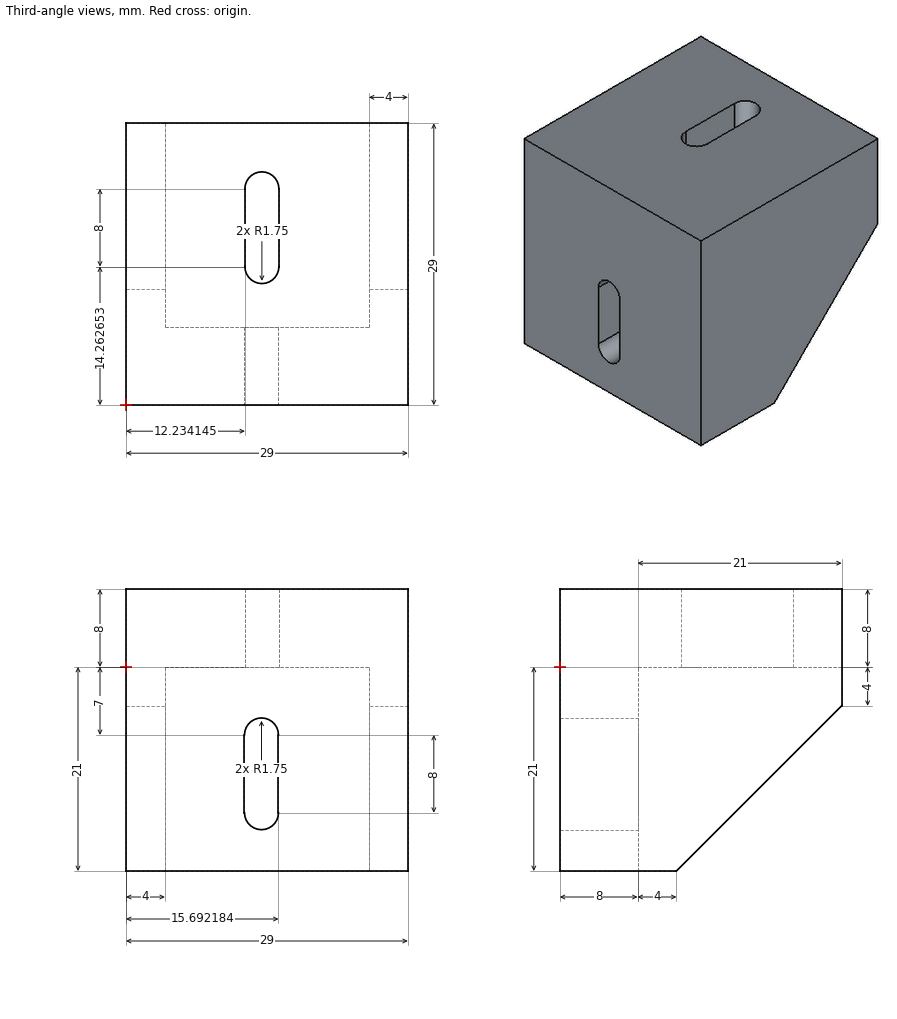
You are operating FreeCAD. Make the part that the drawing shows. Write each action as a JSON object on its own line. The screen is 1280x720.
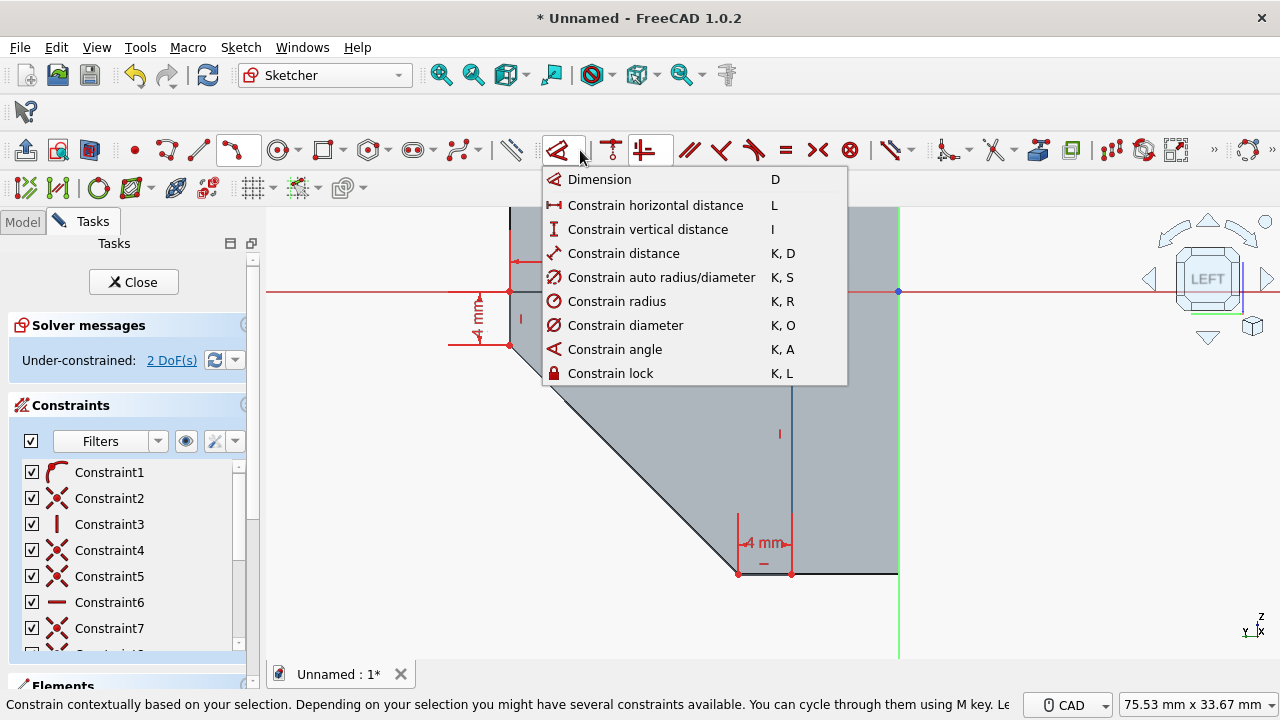
{"action": "left_click", "coordinate": [695, 229]}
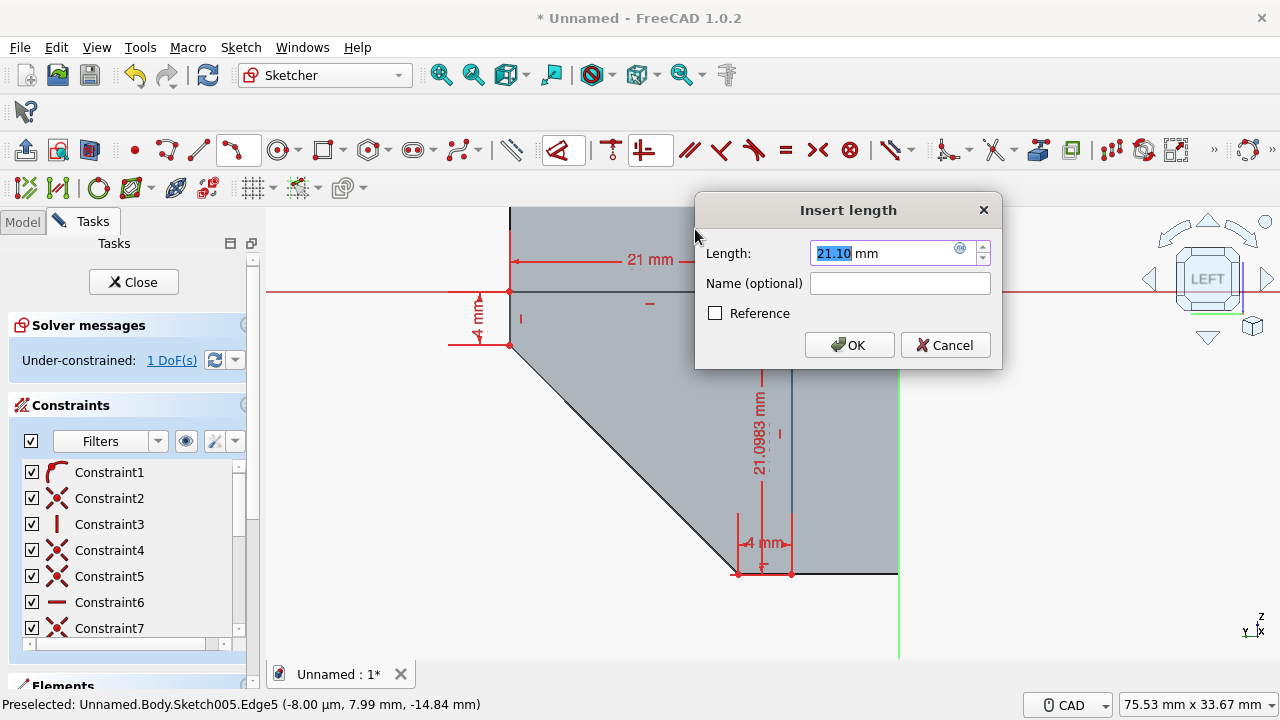
{"action": "type", "text": "21"}
{"action": "key", "text": "Return"}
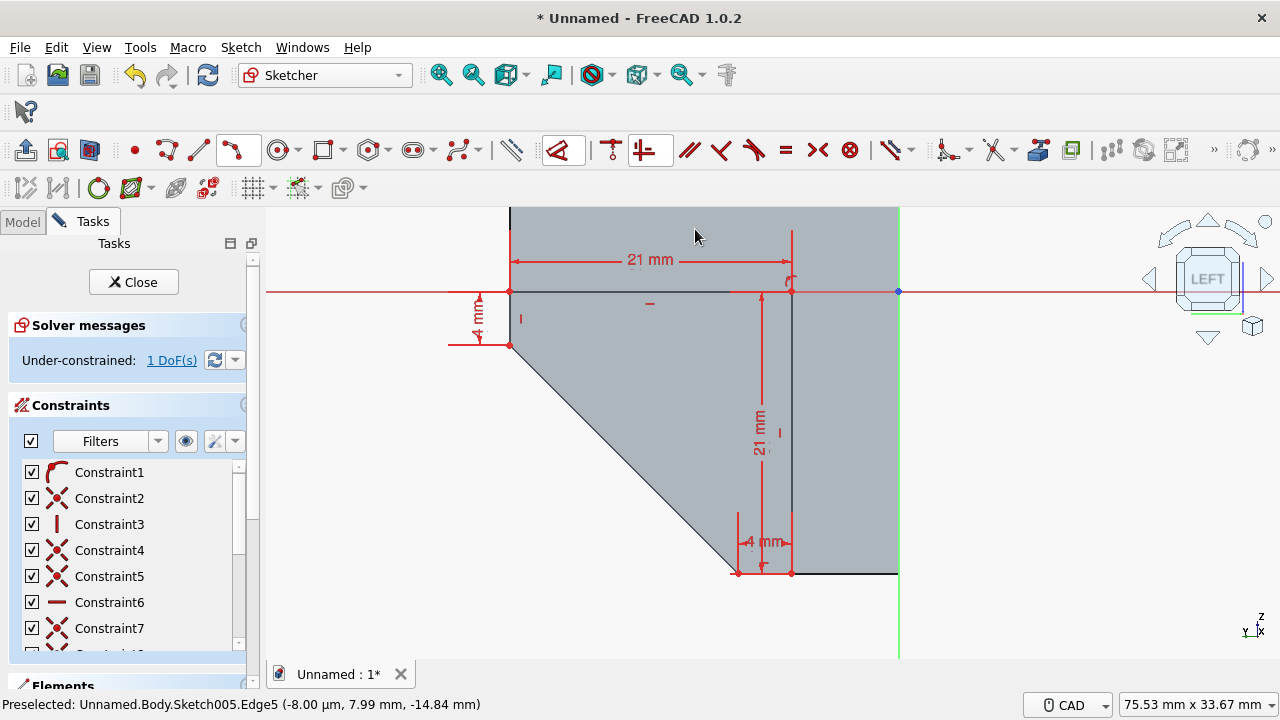
{"action": "left_click", "coordinate": [792, 292]}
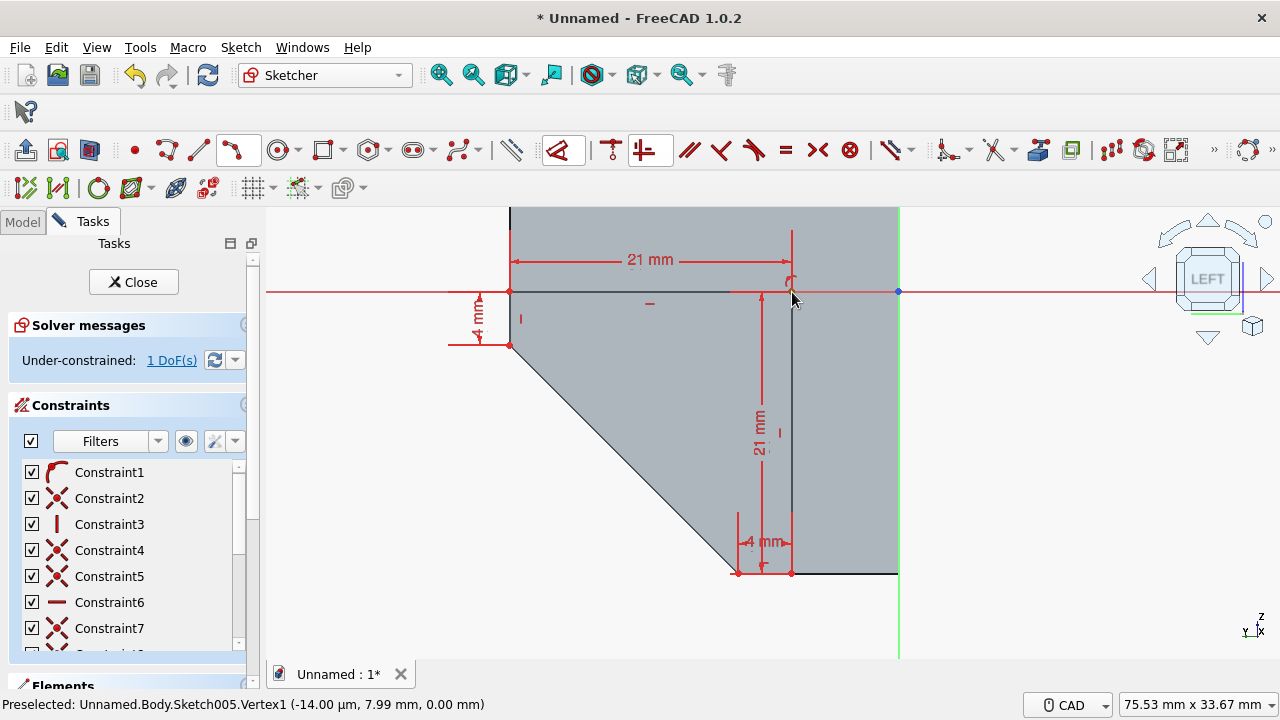
{"action": "left_click", "coordinate": [580, 150]}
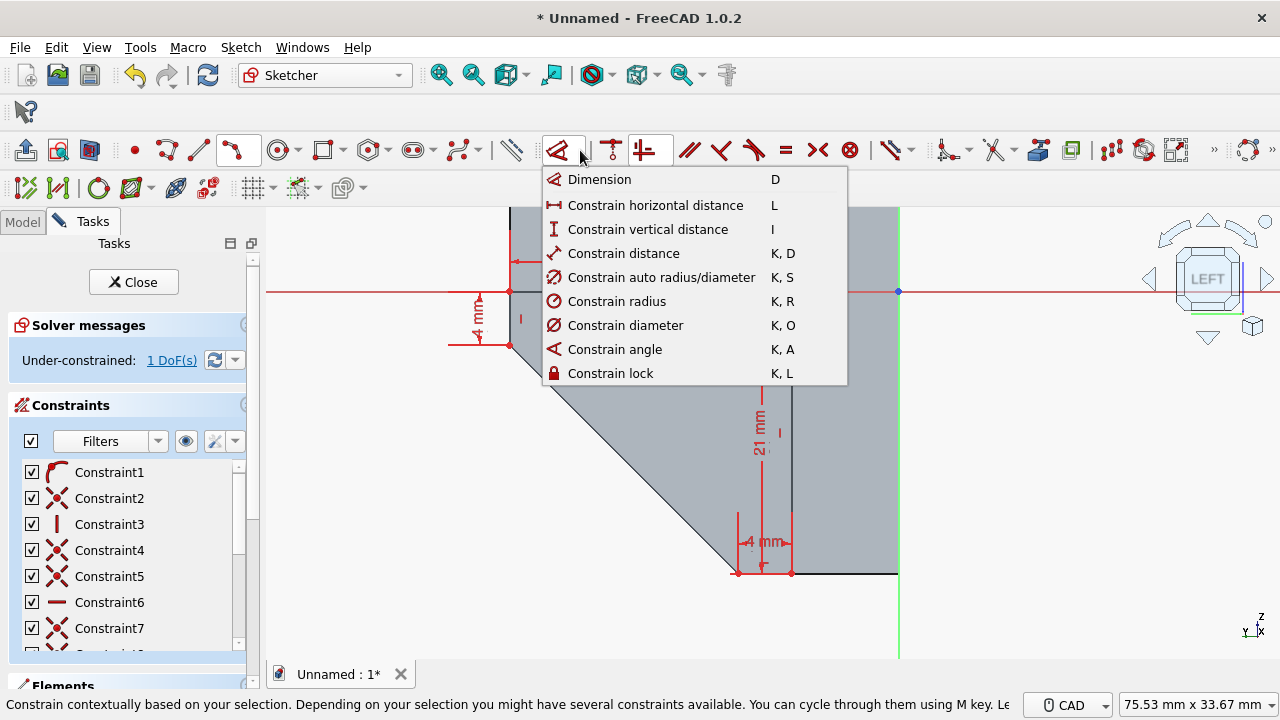
{"action": "left_click", "coordinate": [695, 205]}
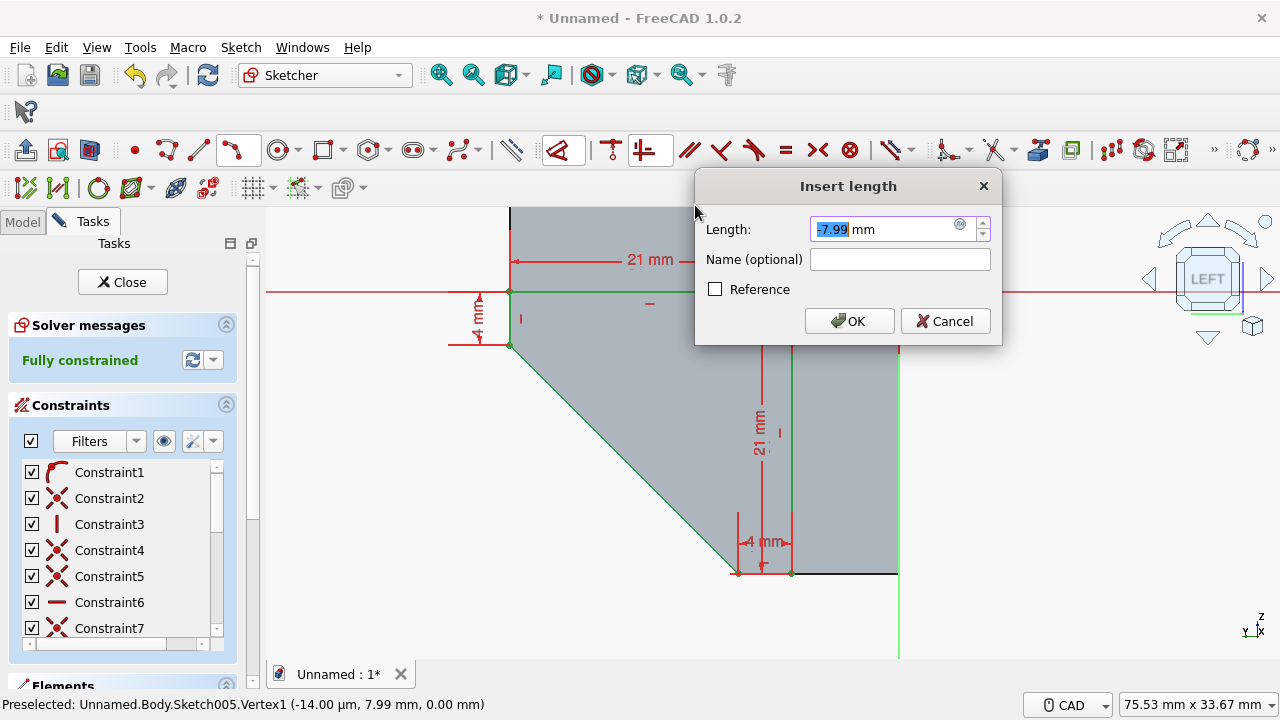
{"action": "type", "text": "-8"}
{"action": "key", "text": "Return"}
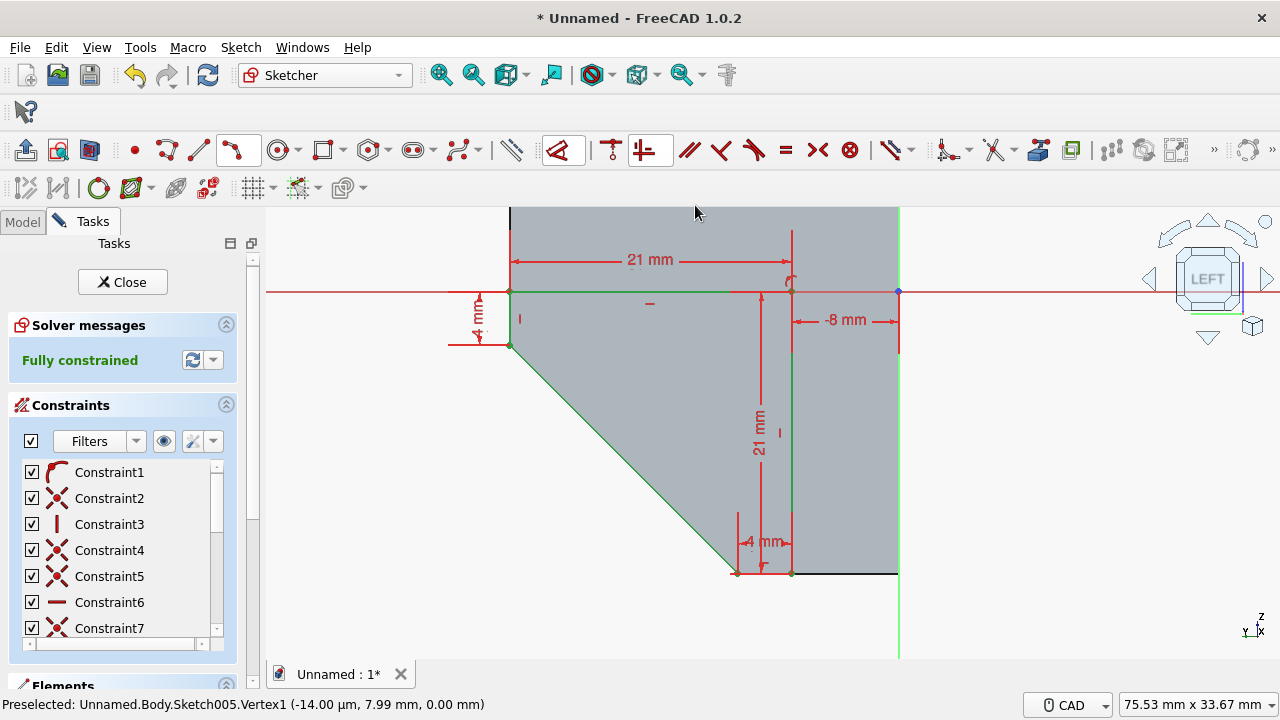
{"action": "left_click", "coordinate": [123, 282]}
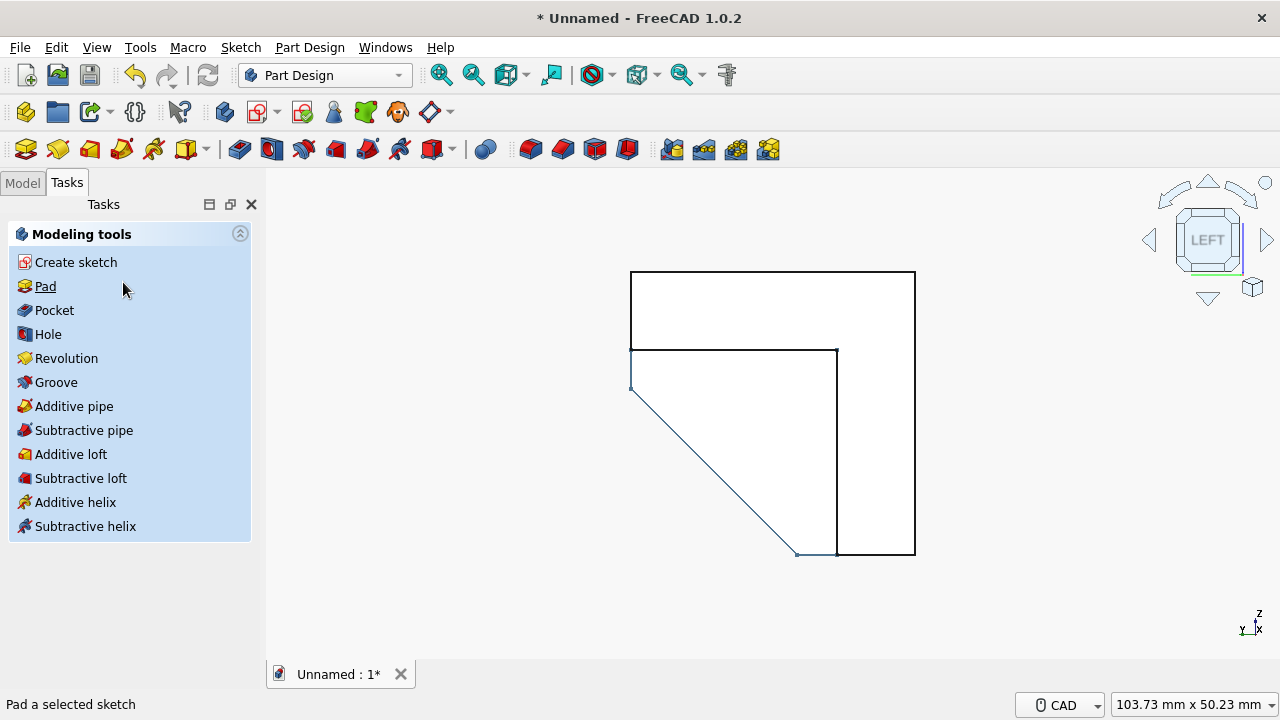
{"action": "left_click", "coordinate": [26, 150]}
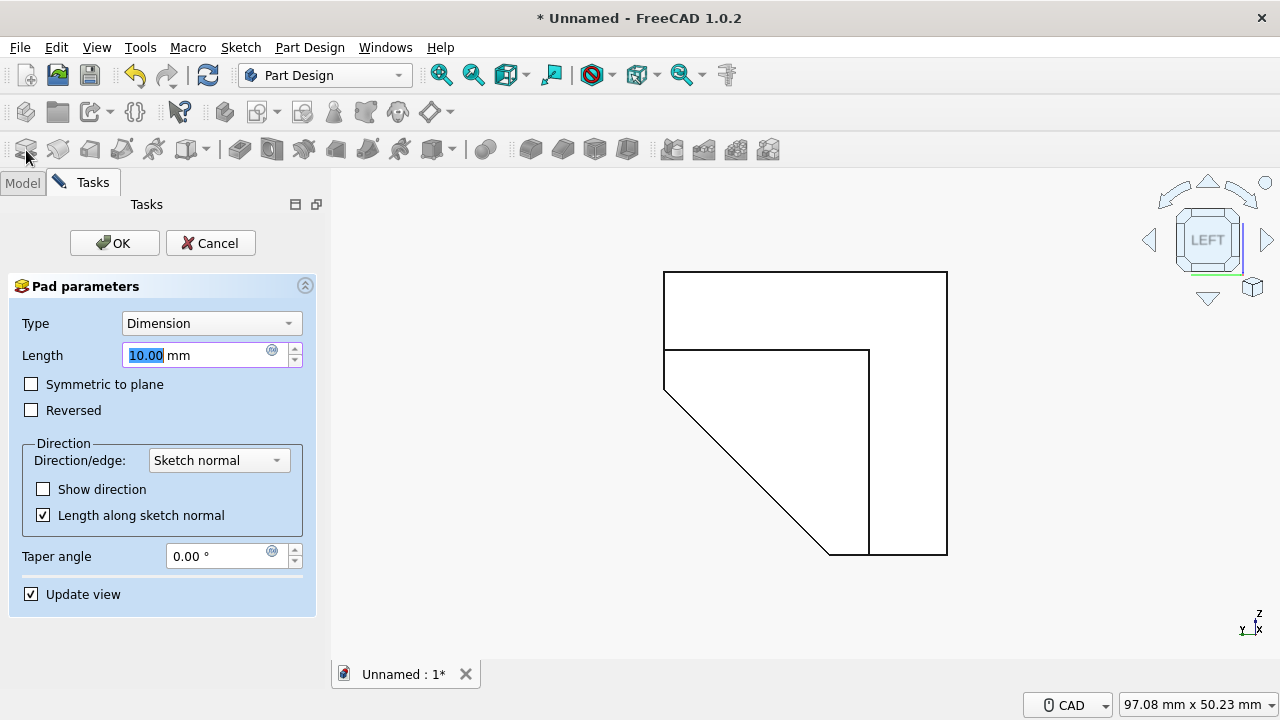
{"action": "type", "text": "4"}
{"action": "key", "text": "Tab"}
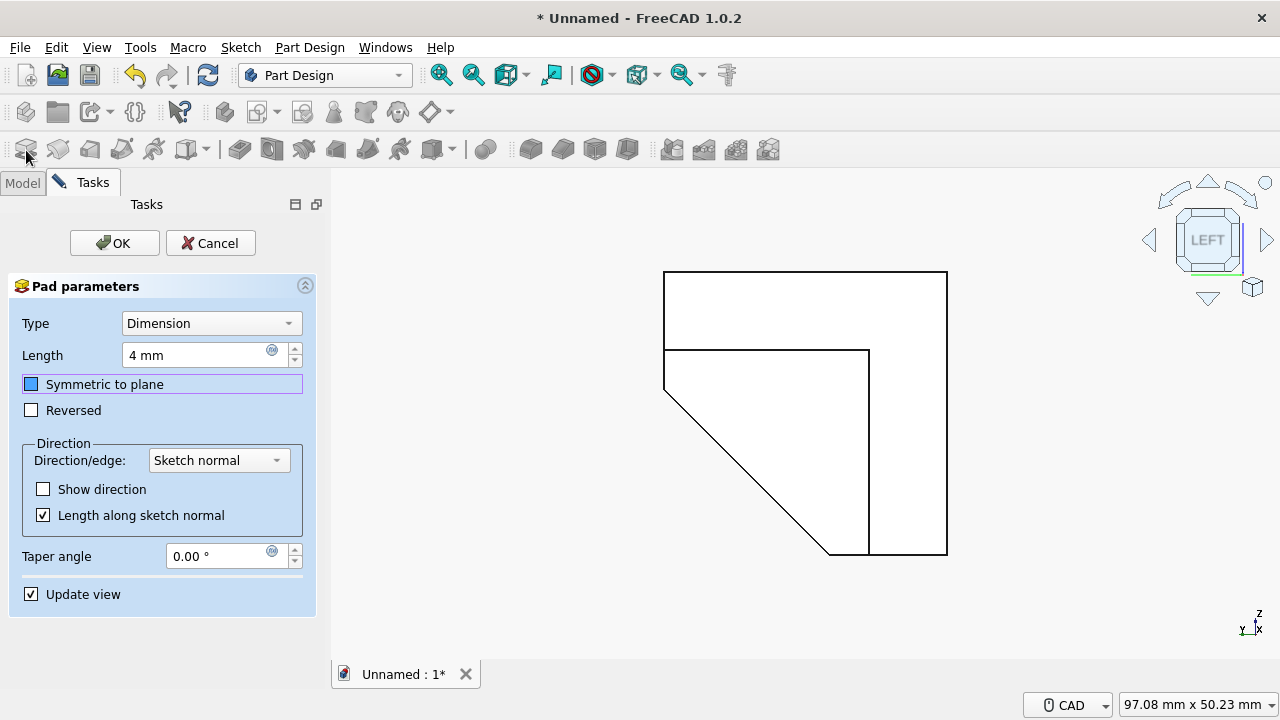
{"action": "left_click", "coordinate": [30, 410]}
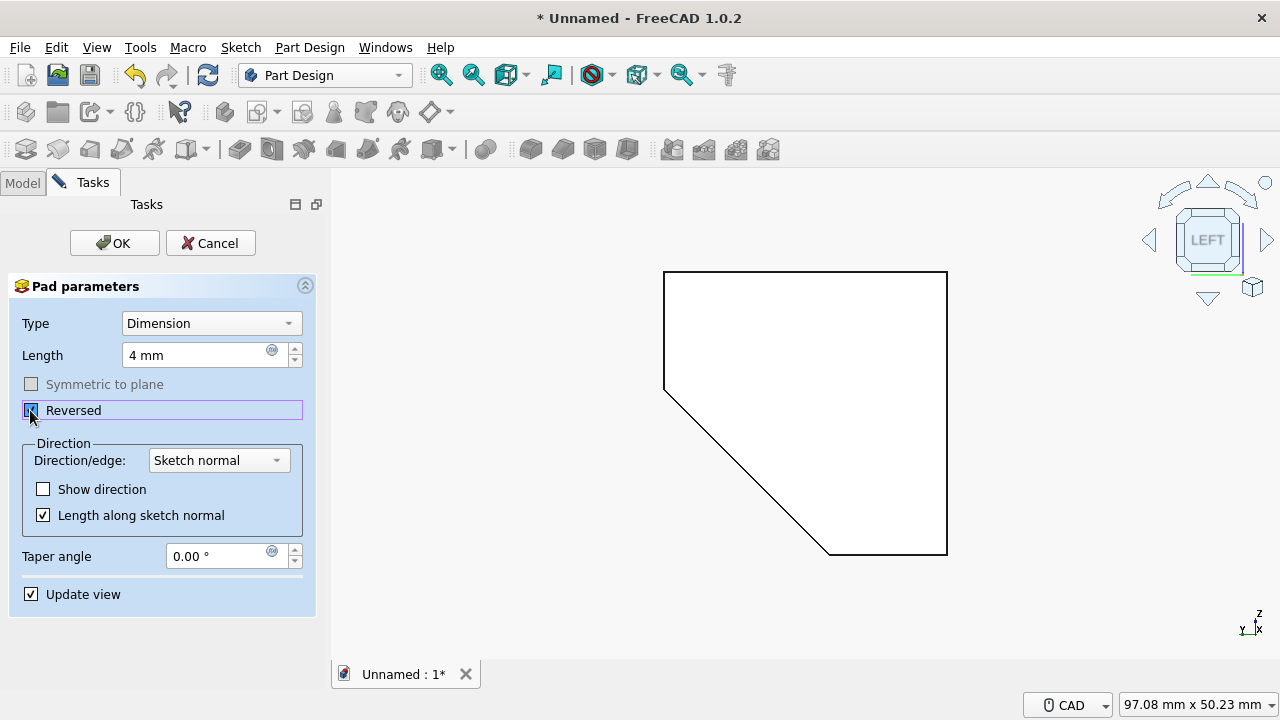
{"action": "left_click", "coordinate": [115, 243]}